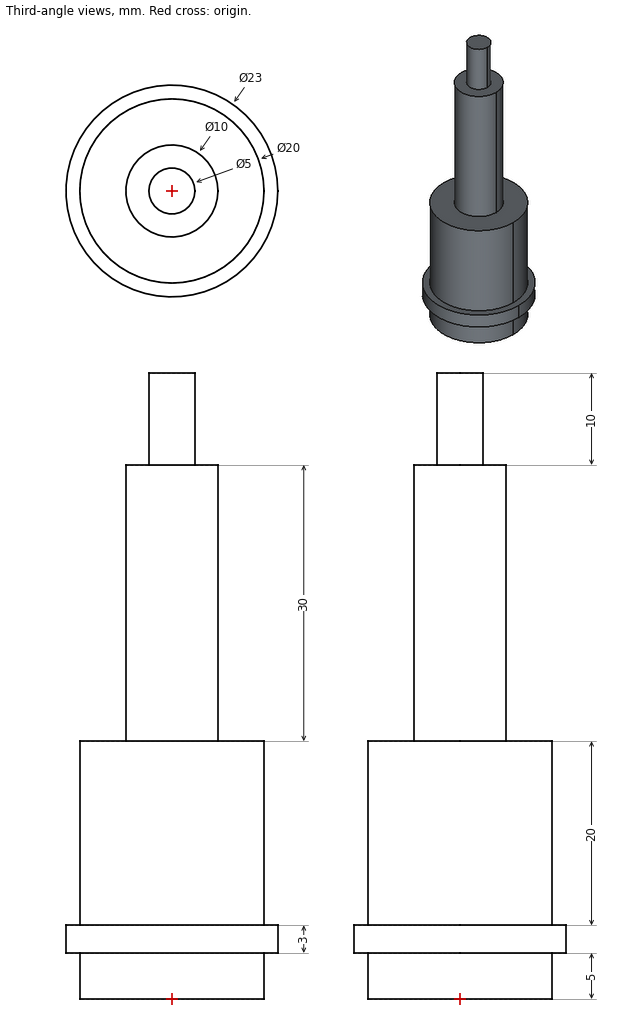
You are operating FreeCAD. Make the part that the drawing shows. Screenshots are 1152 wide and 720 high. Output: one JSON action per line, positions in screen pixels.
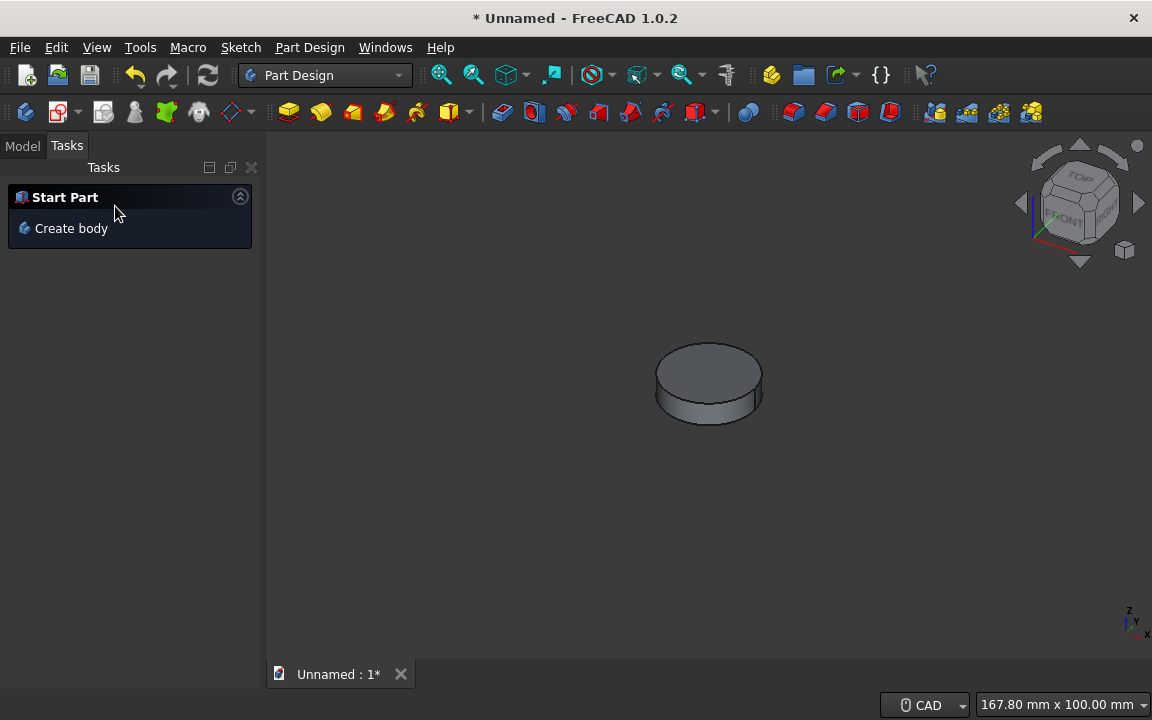
{"action": "left_click", "coordinate": [442, 76]}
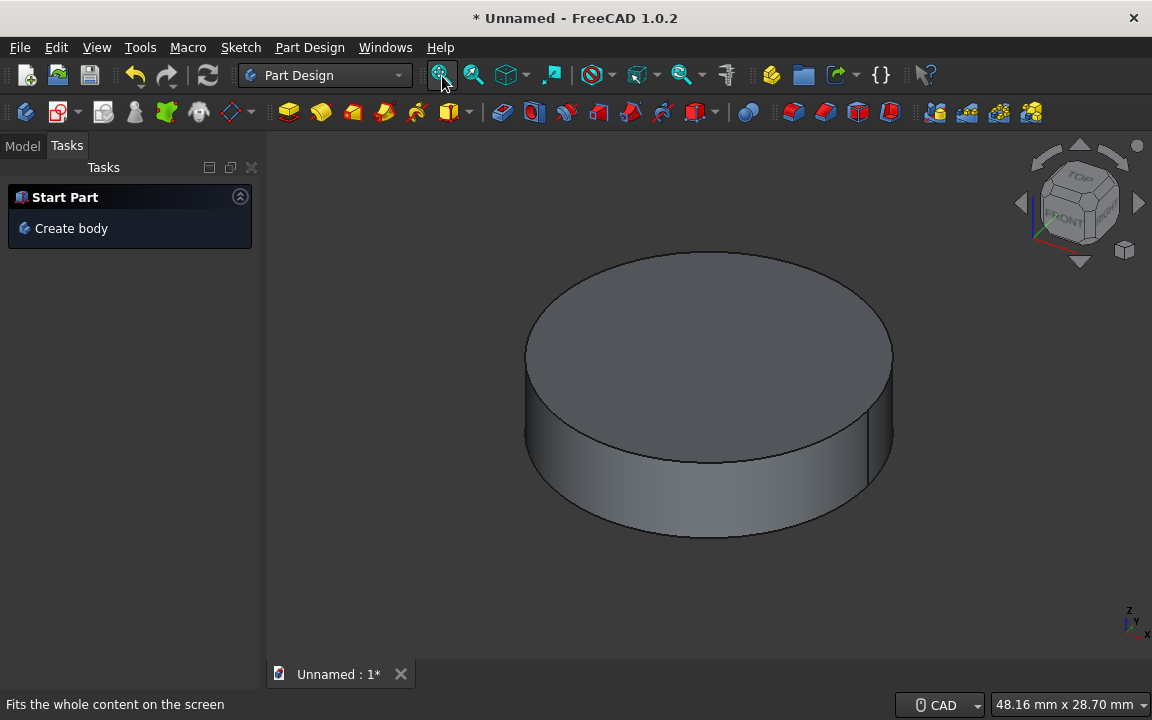
{"action": "left_click", "coordinate": [709, 356]}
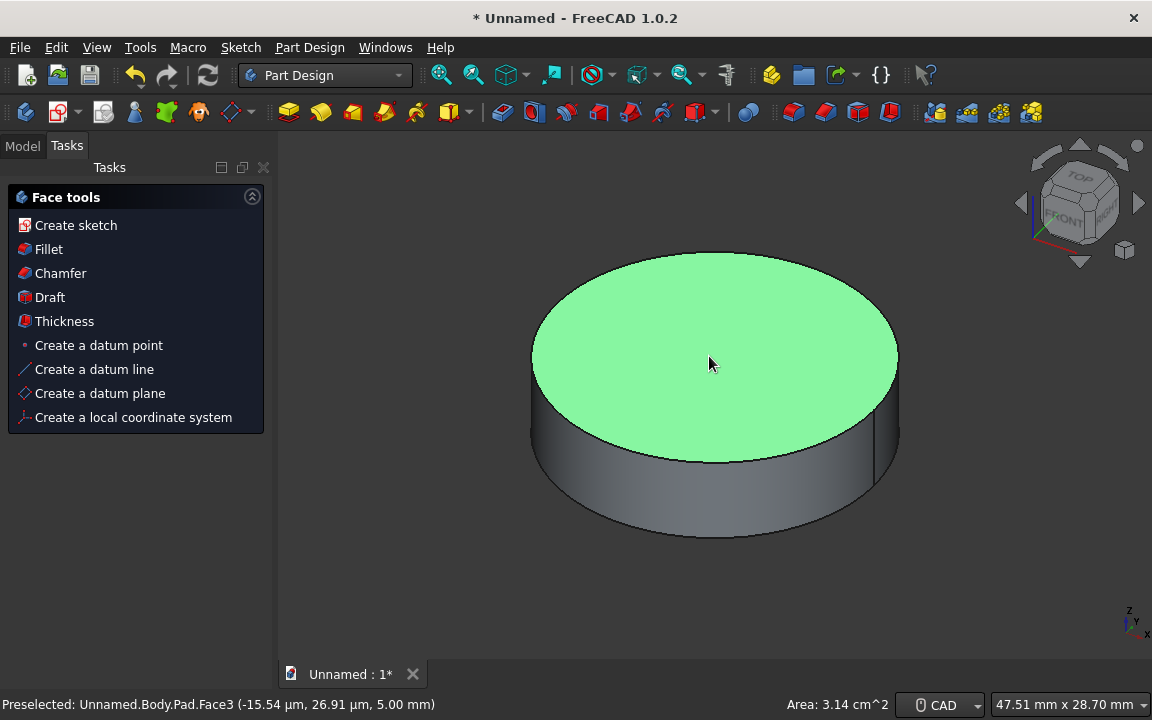
{"action": "left_click", "coordinate": [58, 112]}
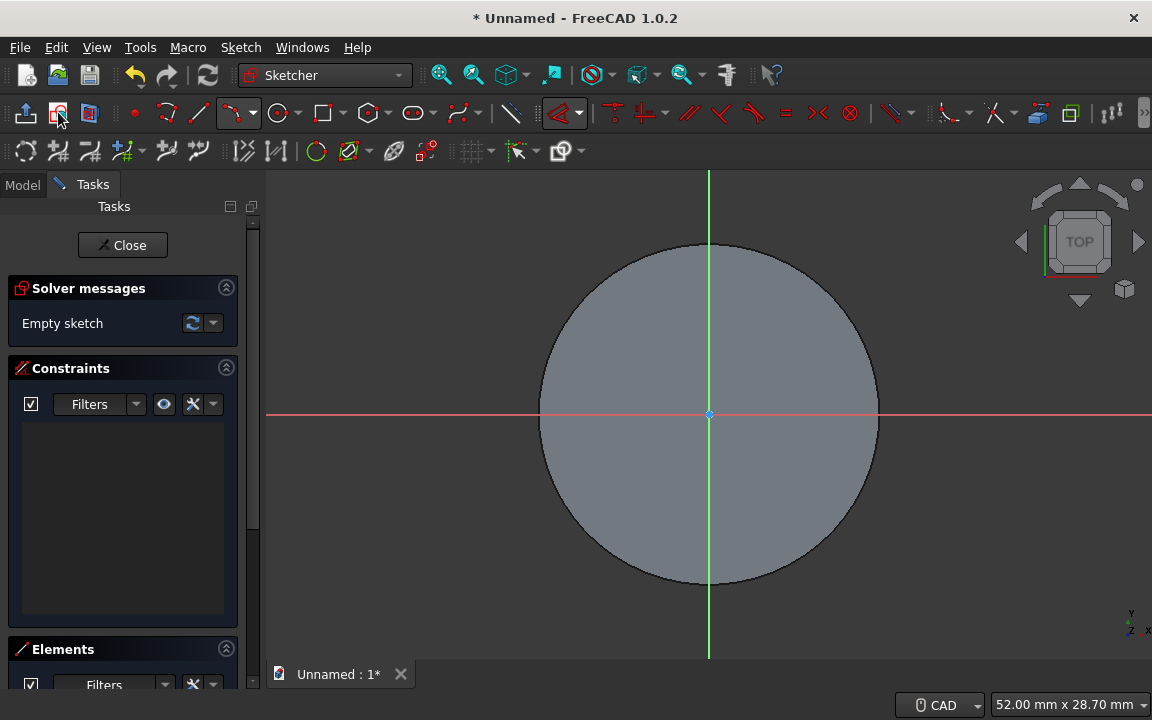
{"action": "scroll", "coordinate": [331, 415], "scroll_direction": "down", "scroll_amount": 1}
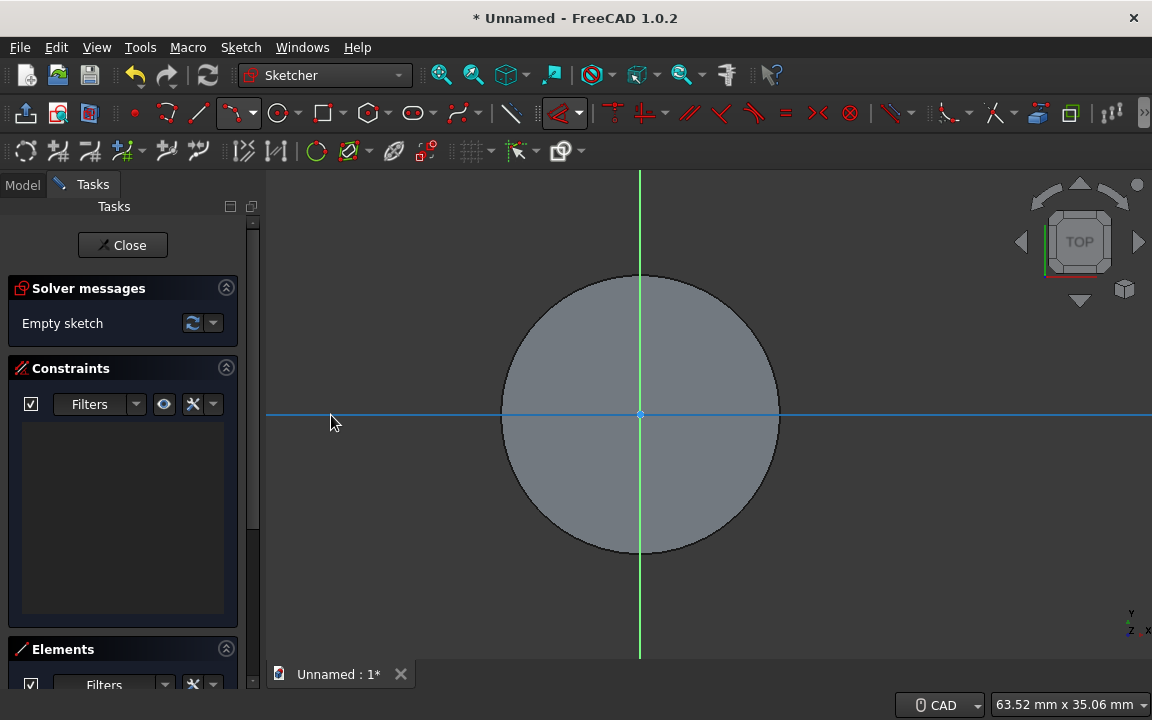
{"action": "left_click", "coordinate": [278, 114]}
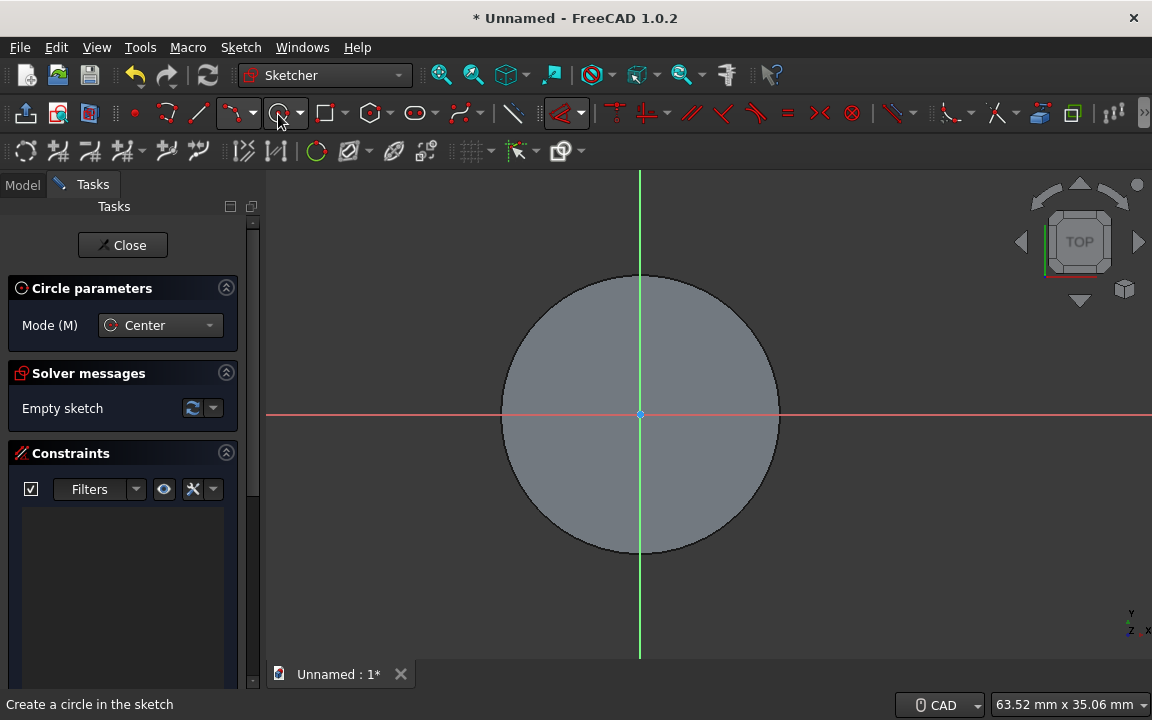
{"action": "left_click", "coordinate": [640, 415]}
{"action": "mouse_move", "coordinate": [754, 301]}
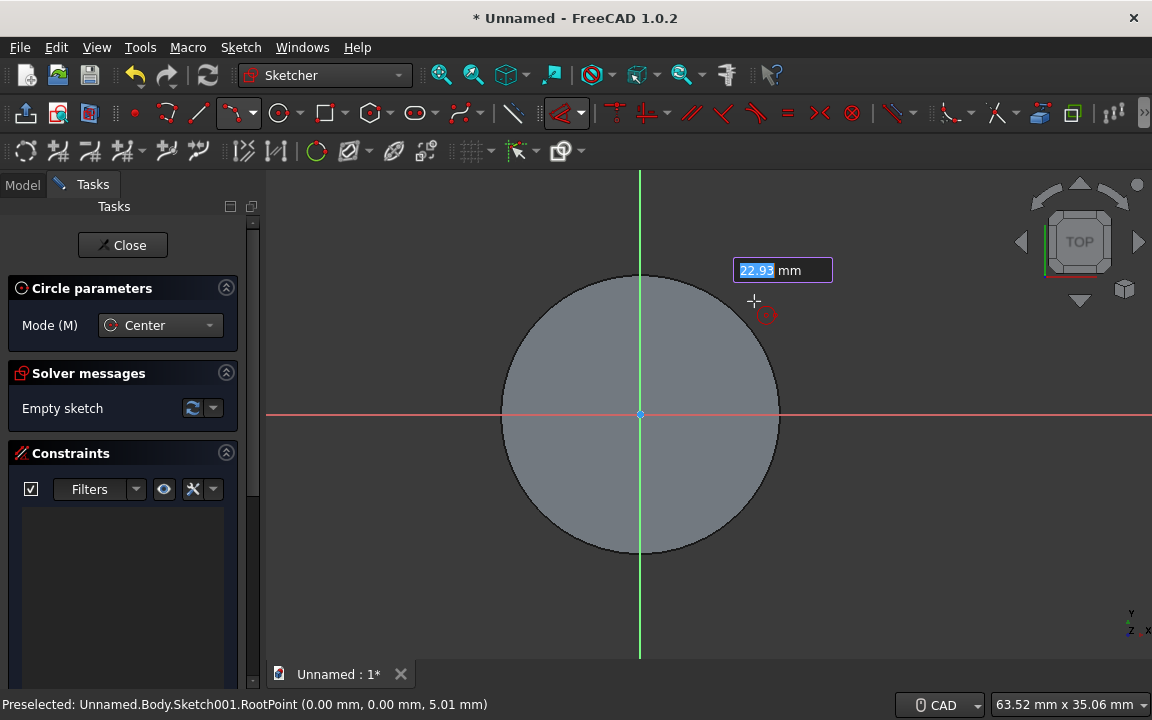
{"action": "type", "text": "23"}
{"action": "key", "text": "Return"}
{"action": "key", "text": "Escape"}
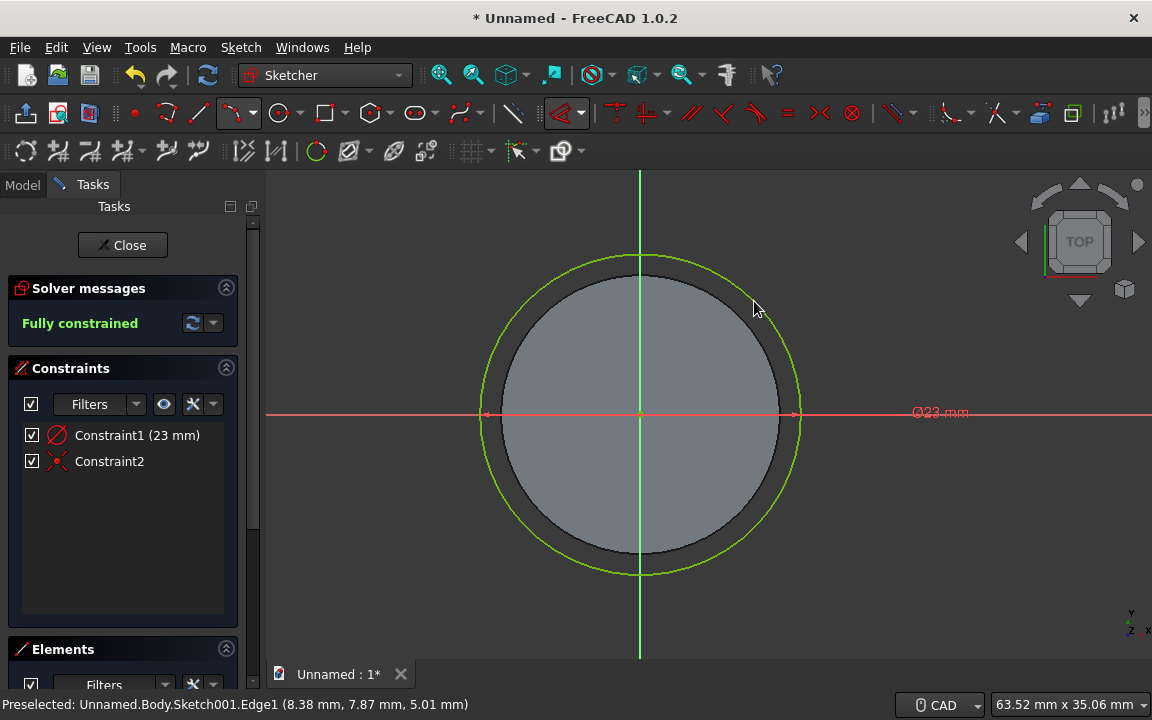
{"action": "left_click", "coordinate": [123, 245]}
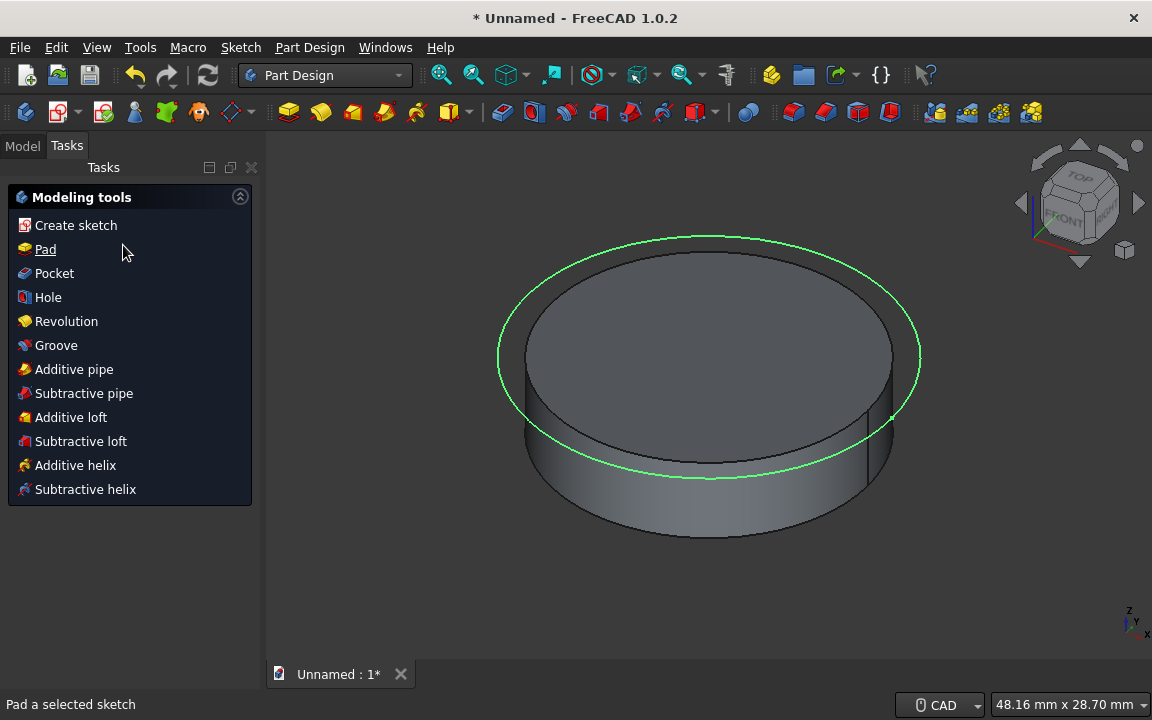
{"action": "left_click", "coordinate": [290, 112]}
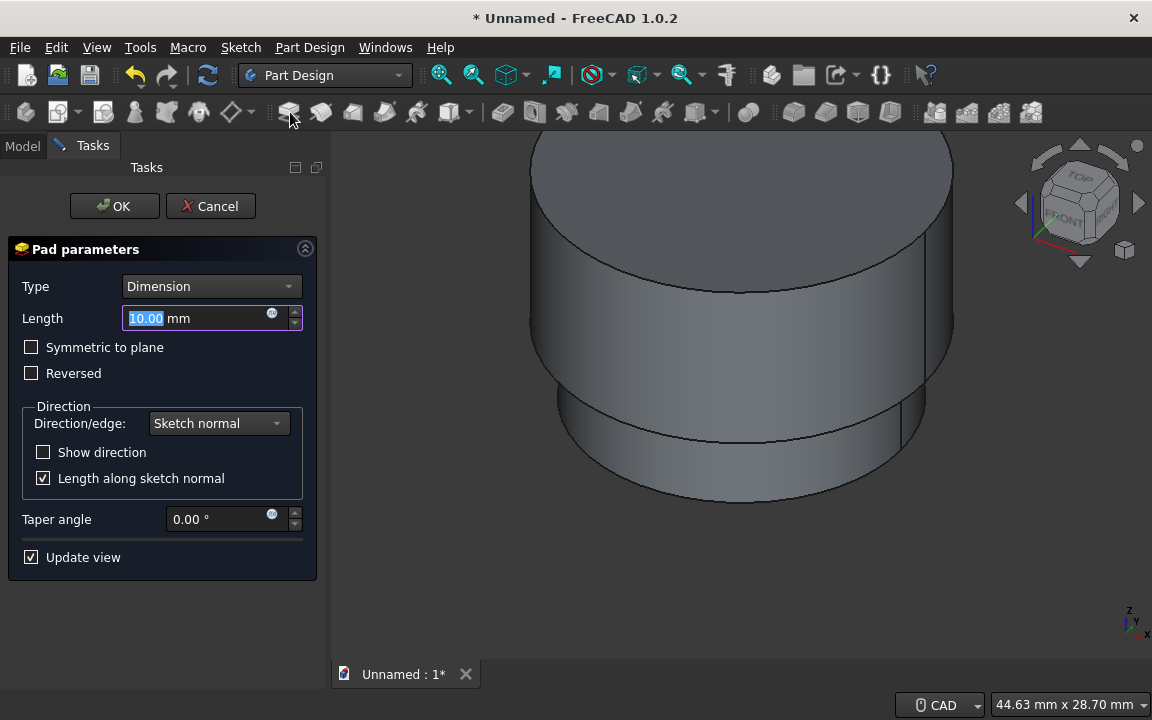
{"action": "type", "text": "3"}
{"action": "key", "text": "Tab"}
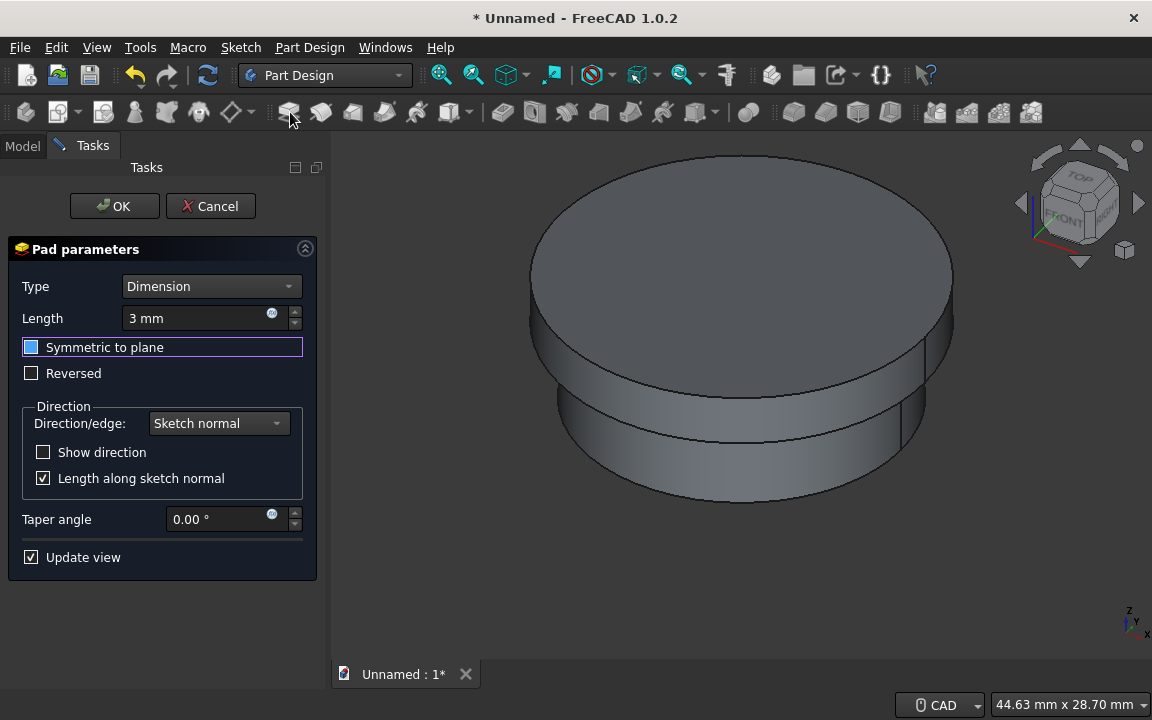
{"action": "left_click", "coordinate": [115, 206]}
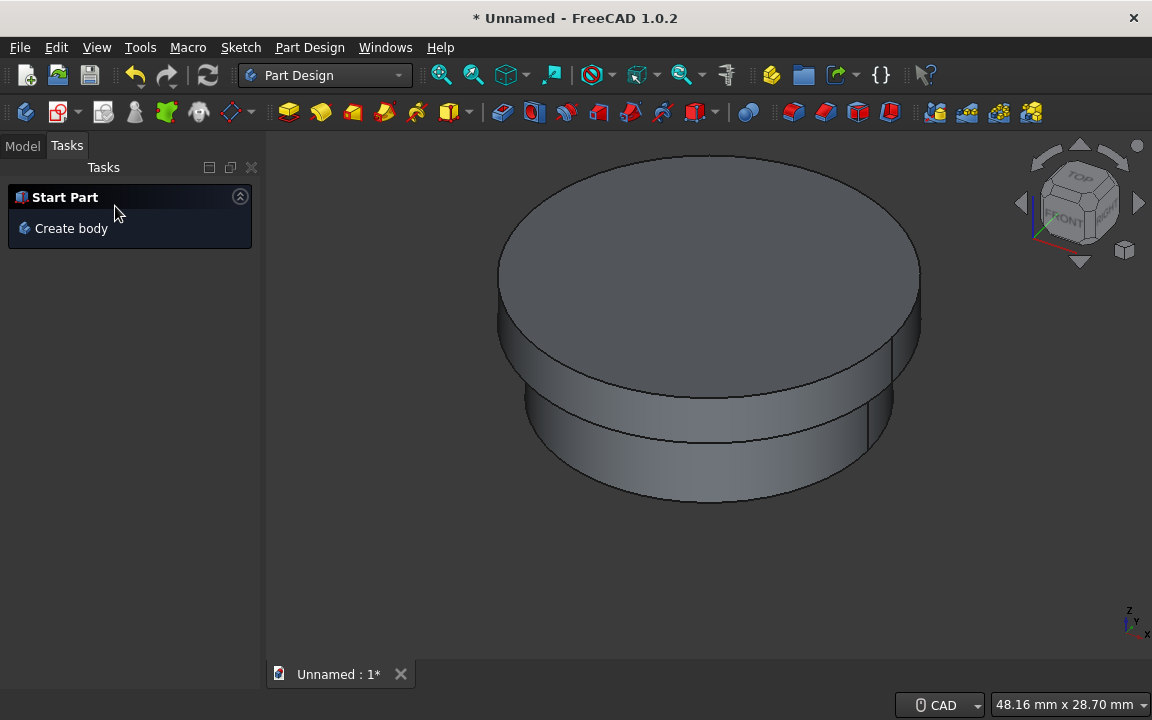
{"action": "left_click", "coordinate": [442, 76]}